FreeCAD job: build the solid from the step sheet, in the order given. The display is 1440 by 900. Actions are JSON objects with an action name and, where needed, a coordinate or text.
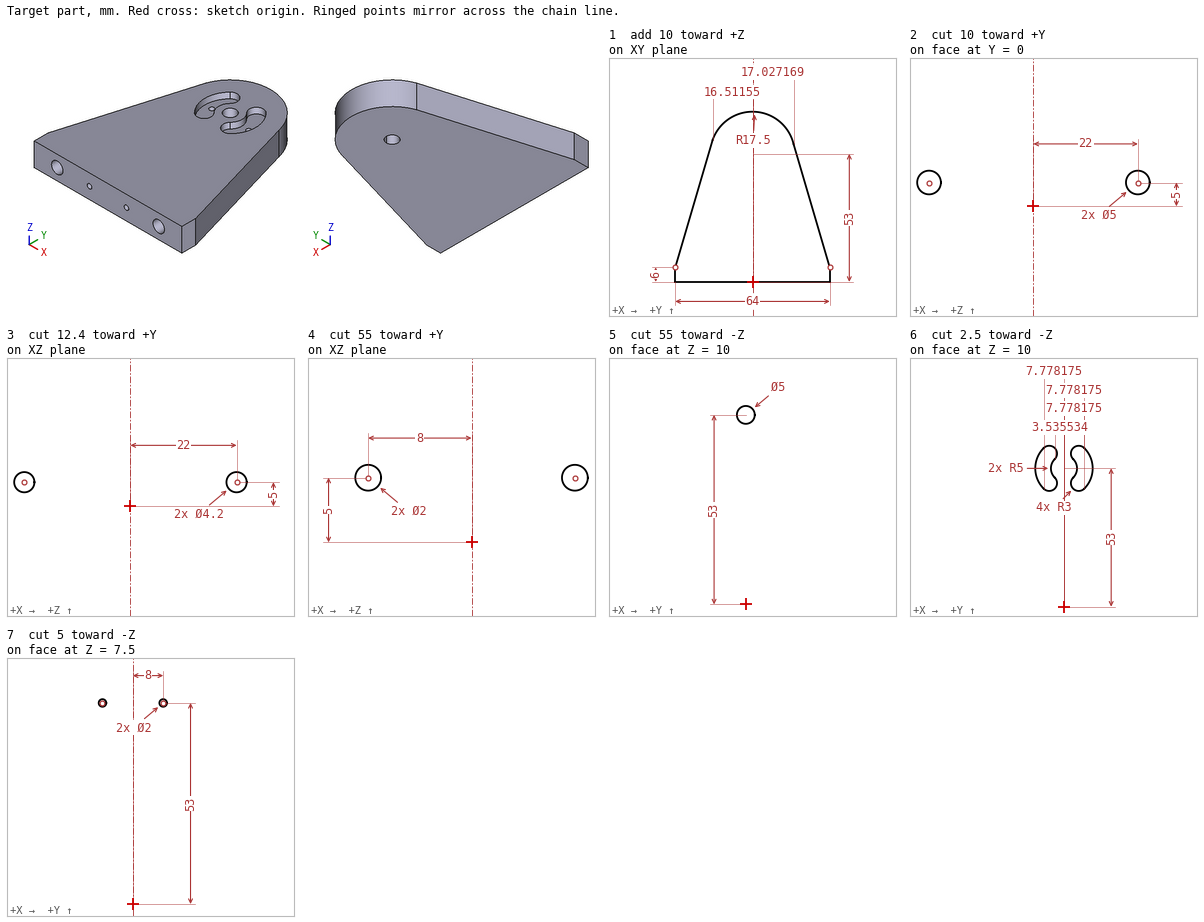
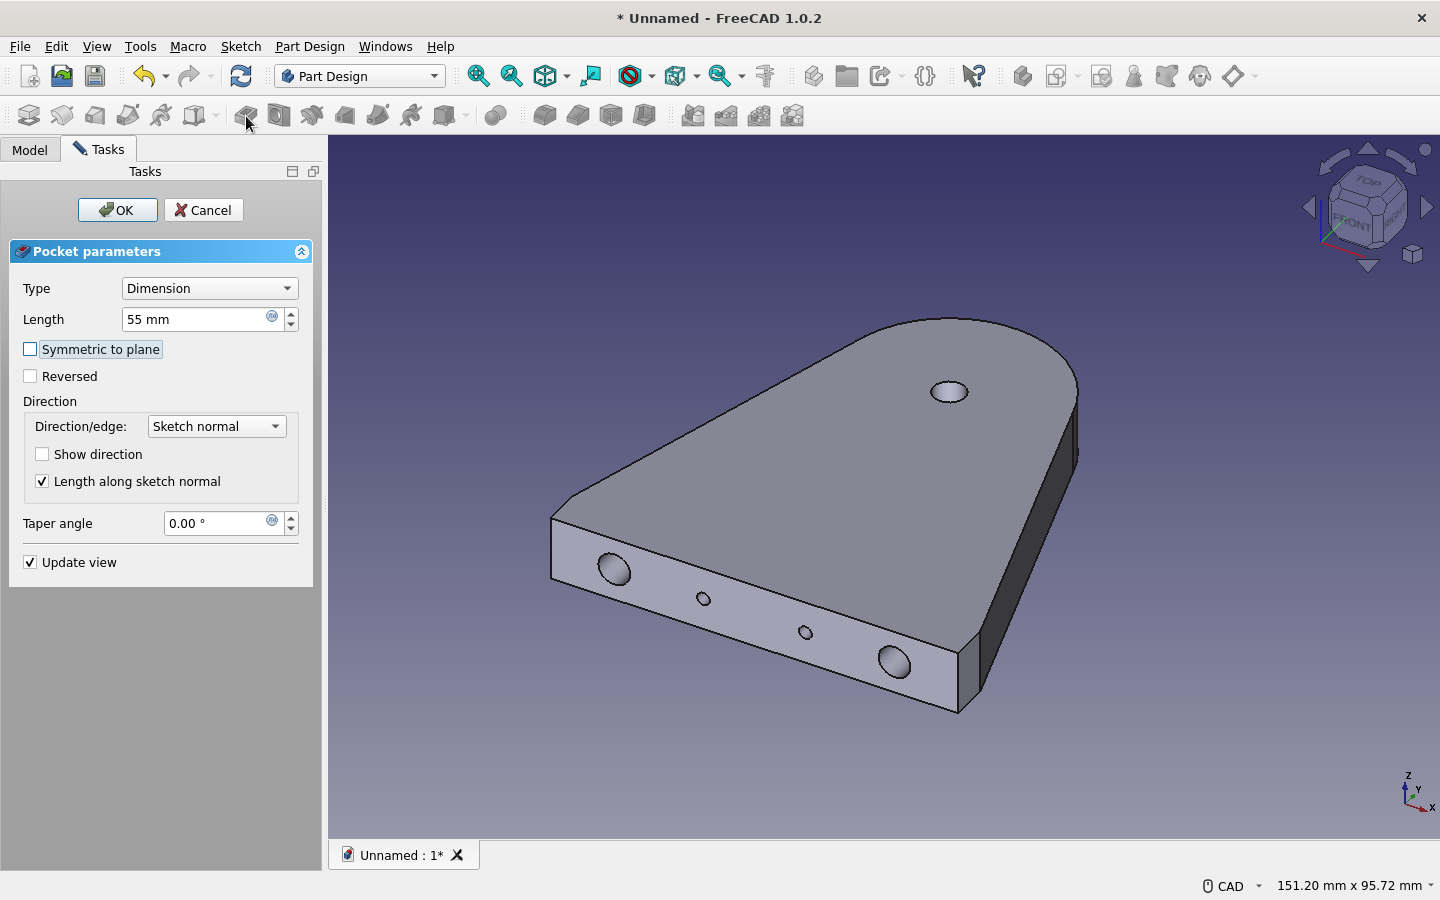
{"action": "left_click", "coordinate": [118, 210]}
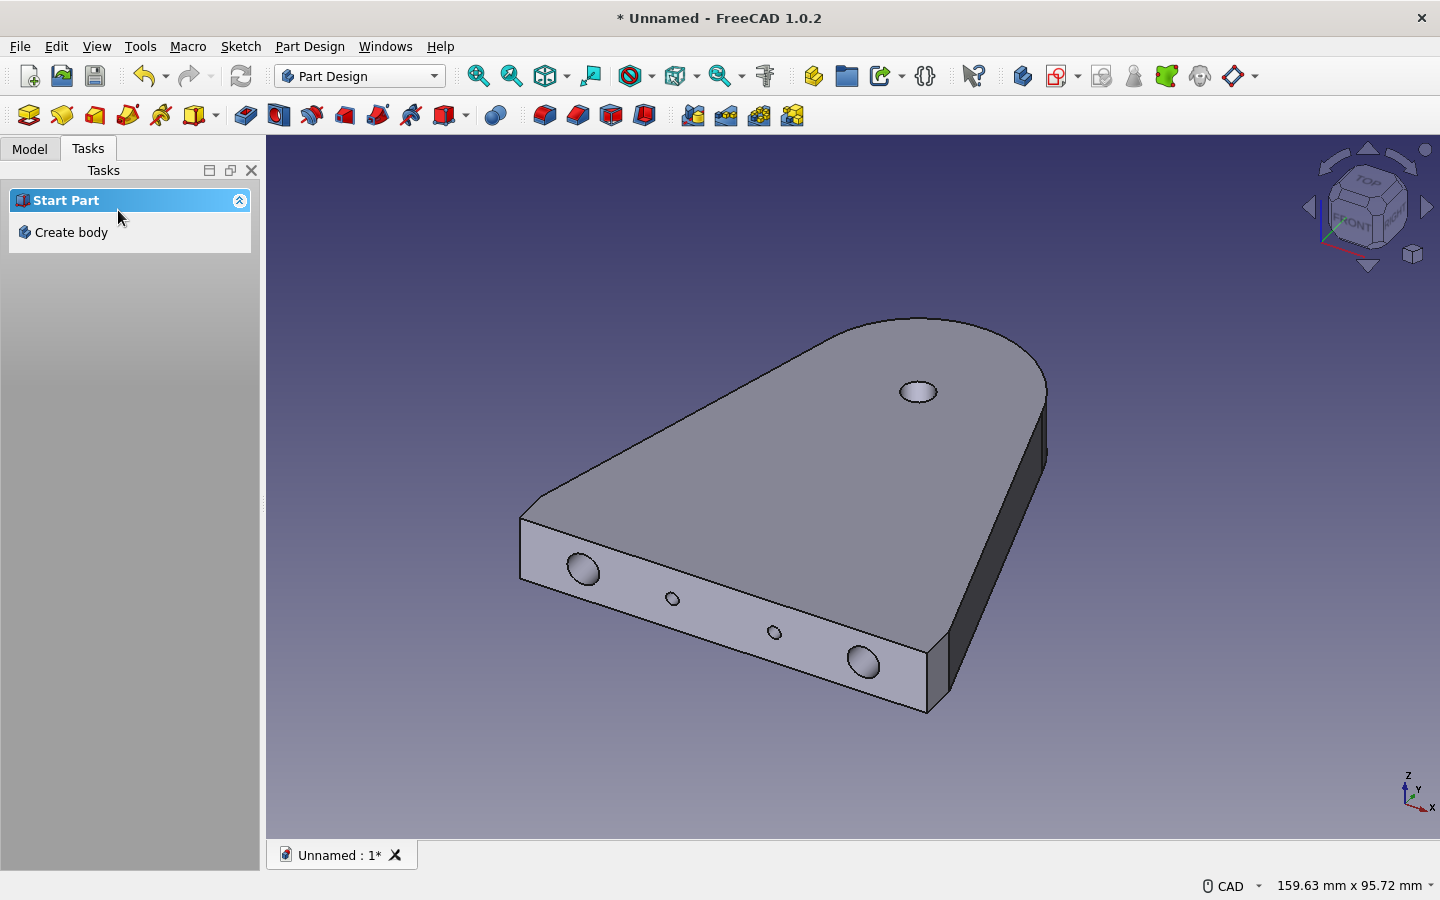
{"action": "left_click", "coordinate": [816, 493]}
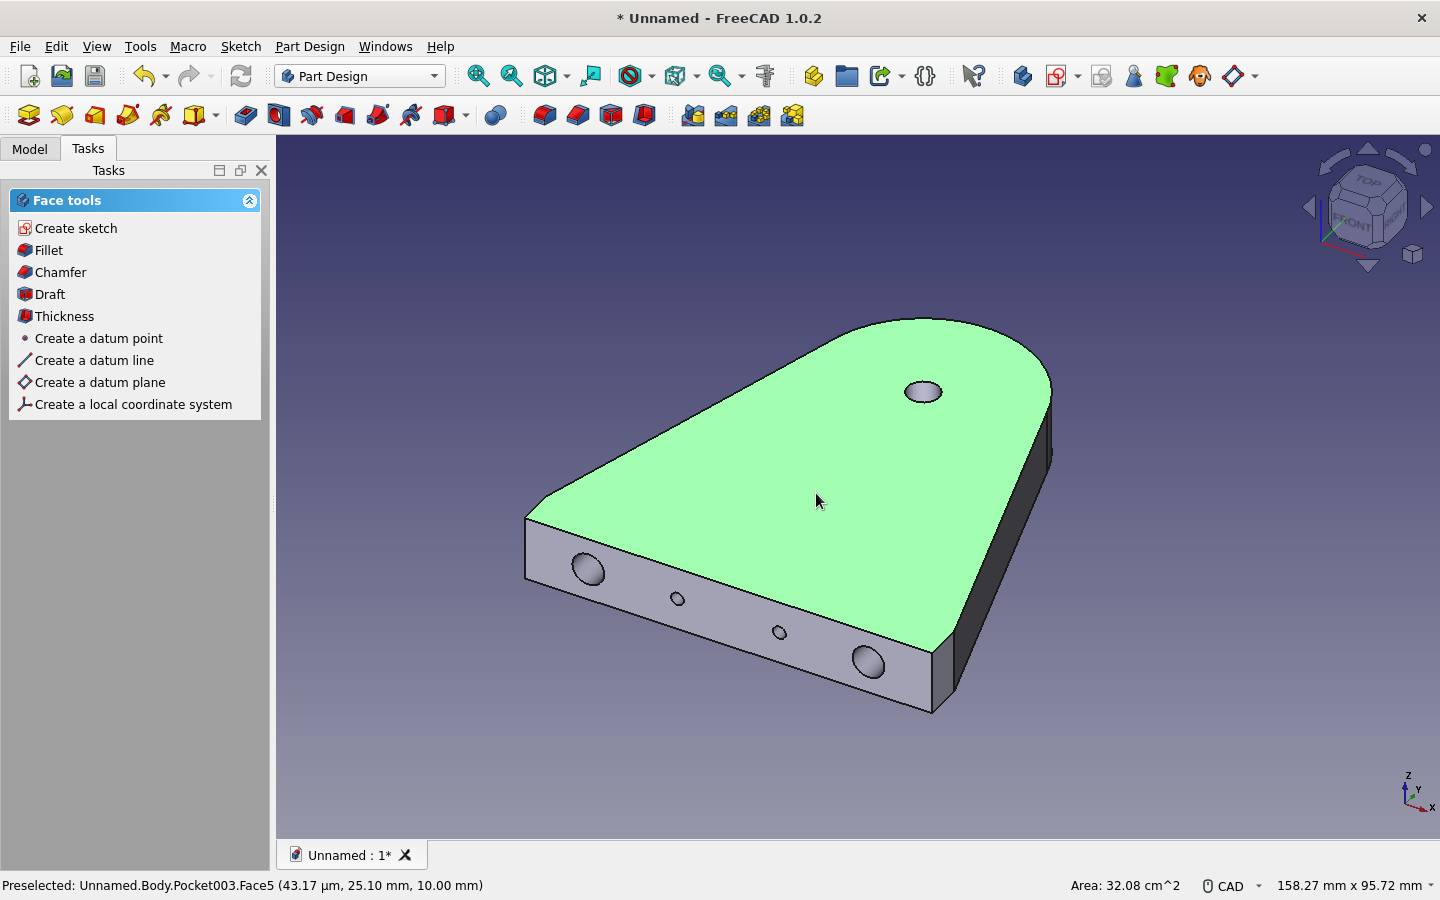
{"action": "left_click", "coordinate": [1056, 76]}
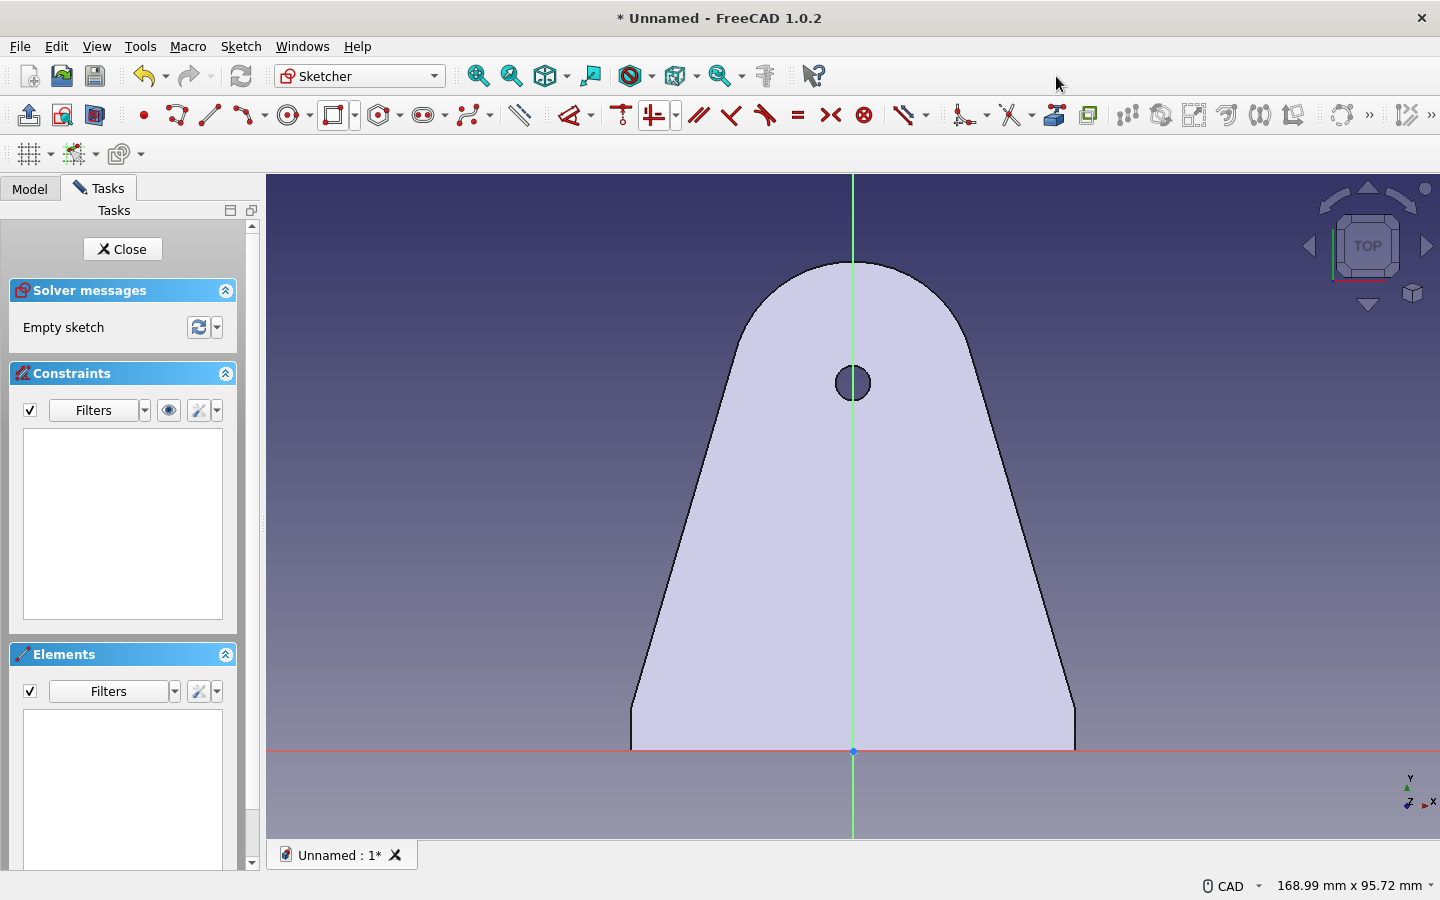
{"action": "scroll", "coordinate": [875, 343], "scroll_direction": "up", "scroll_amount": 7}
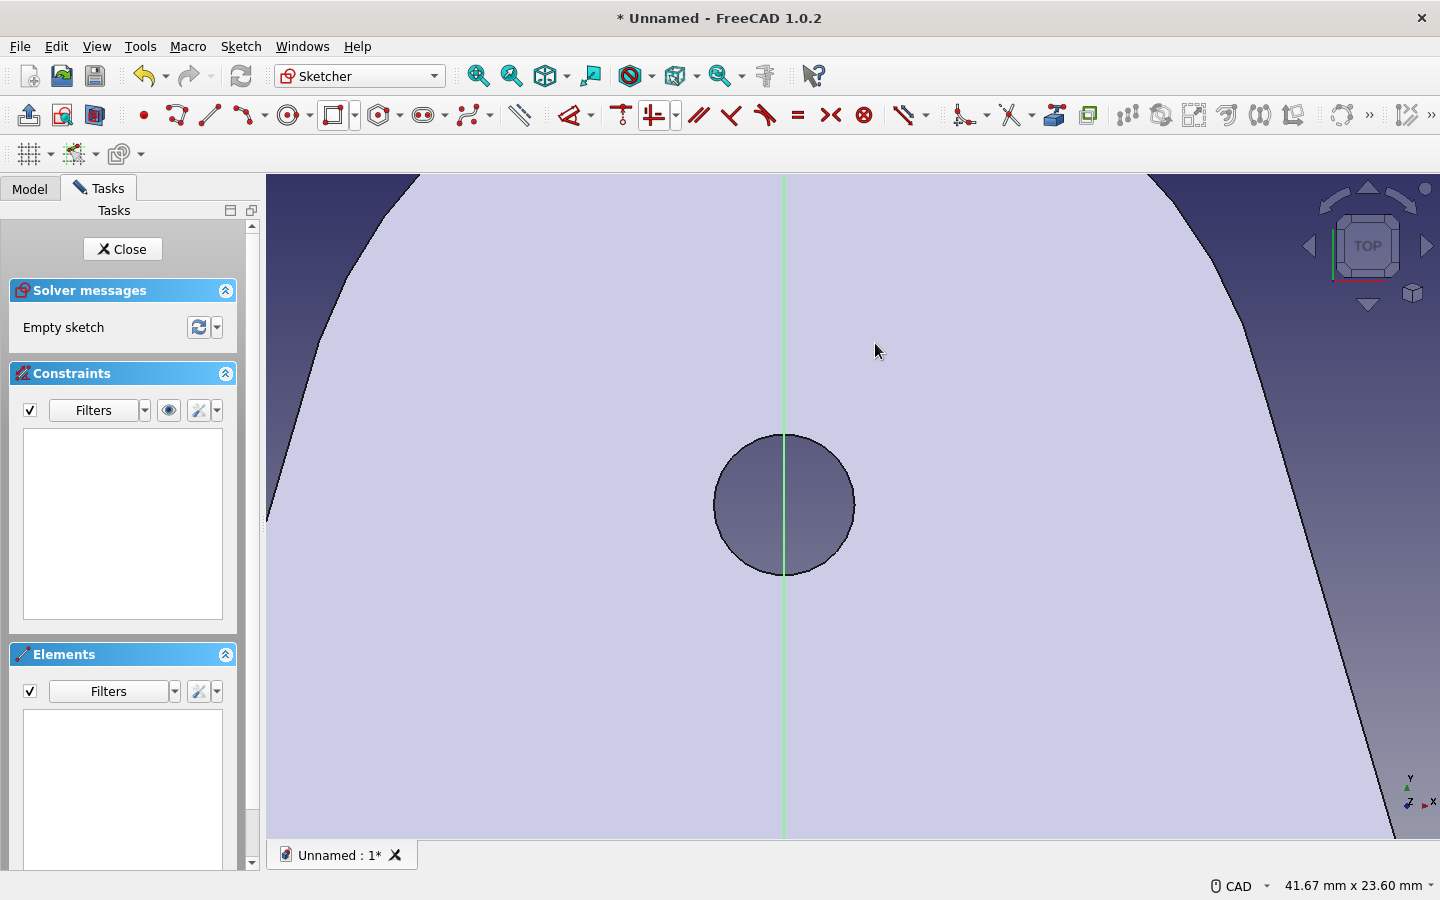
{"action": "left_click", "coordinate": [242, 116]}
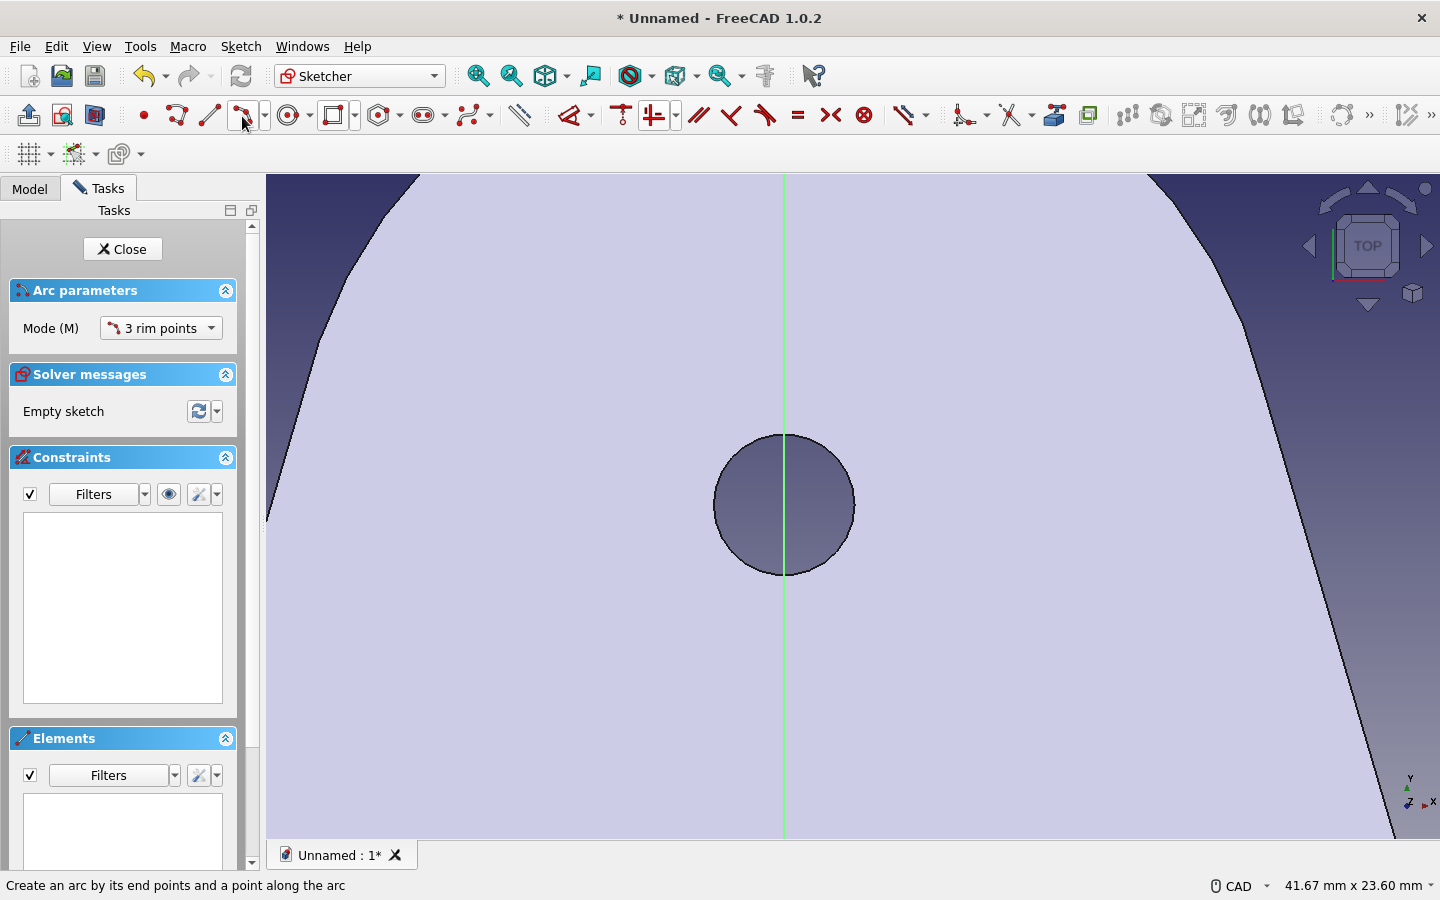
{"action": "left_click", "coordinate": [565, 724]}
{"action": "left_click", "coordinate": [685, 604]}
{"action": "left_click", "coordinate": [685, 724]}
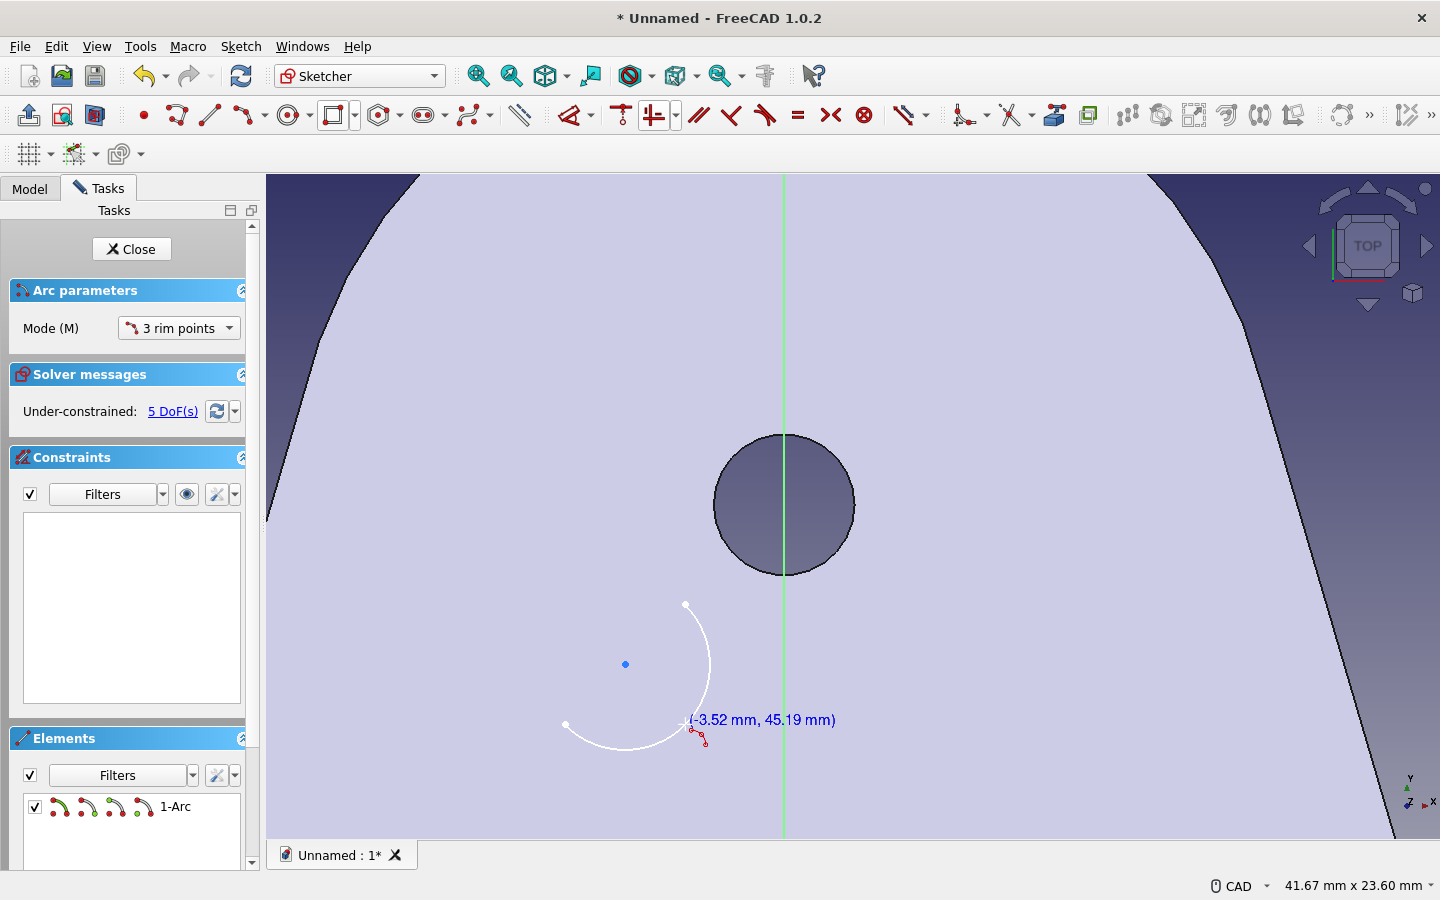
{"action": "left_click", "coordinate": [685, 605]}
{"action": "left_click", "coordinate": [685, 405]}
{"action": "left_click", "coordinate": [643, 505]}